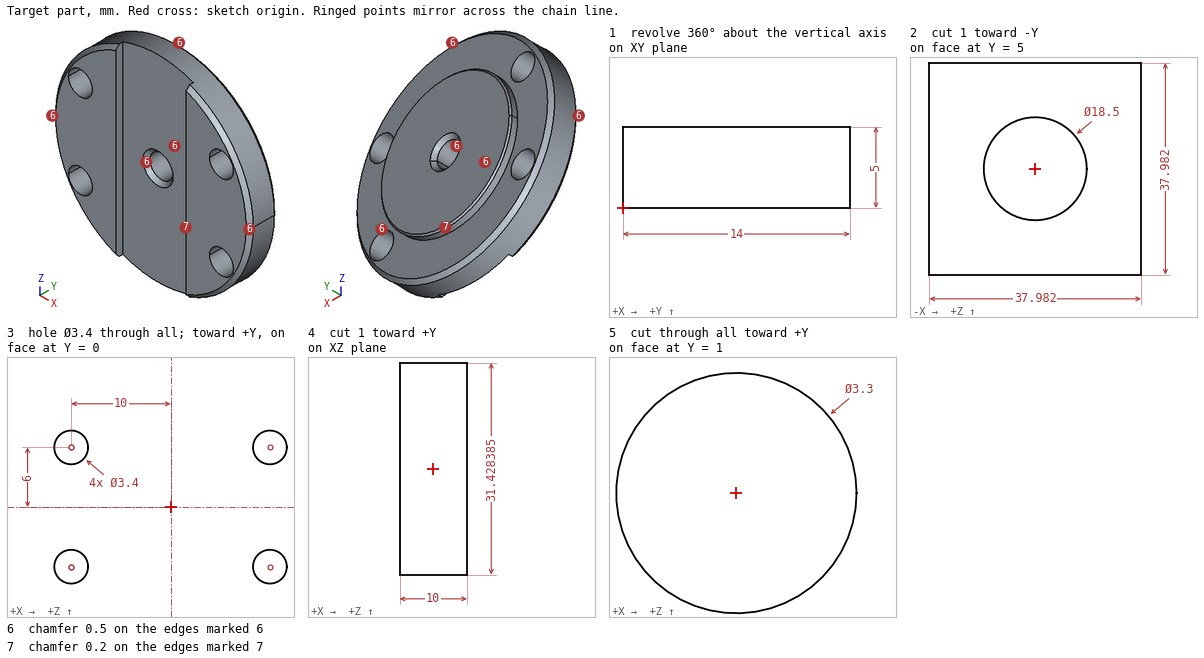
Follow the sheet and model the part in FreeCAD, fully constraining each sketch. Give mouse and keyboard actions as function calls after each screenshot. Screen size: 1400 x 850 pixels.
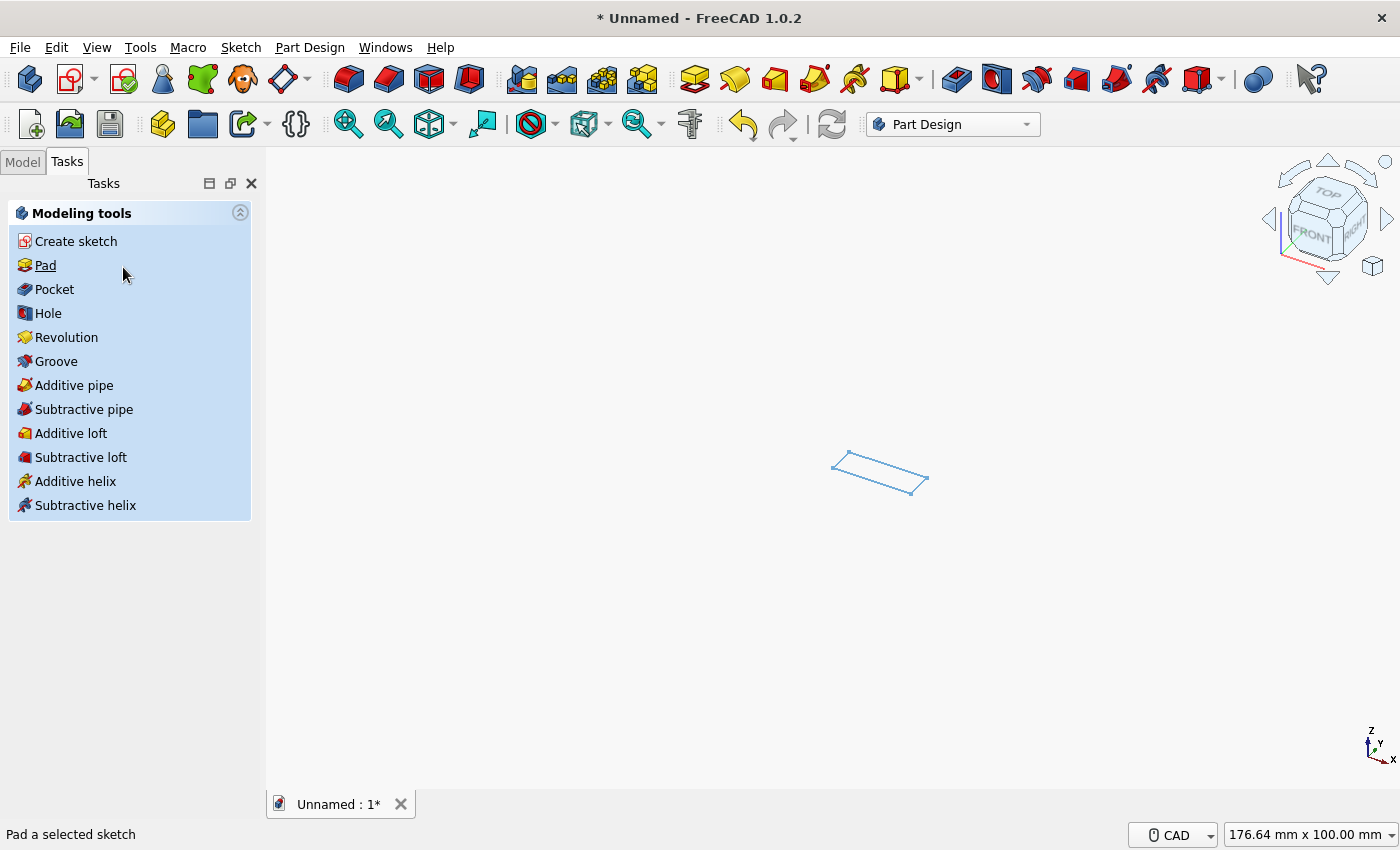
click(736, 80)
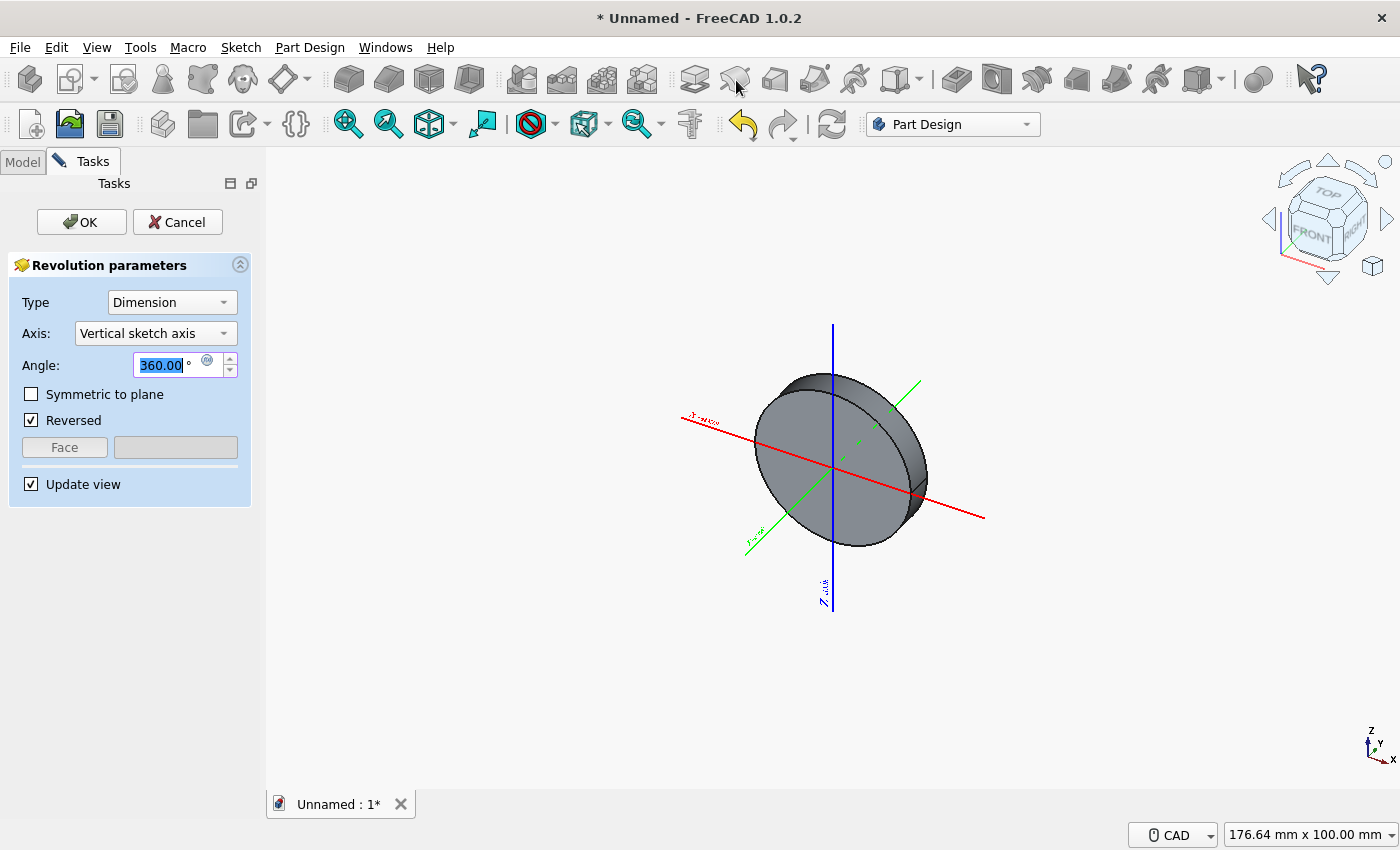
click(82, 222)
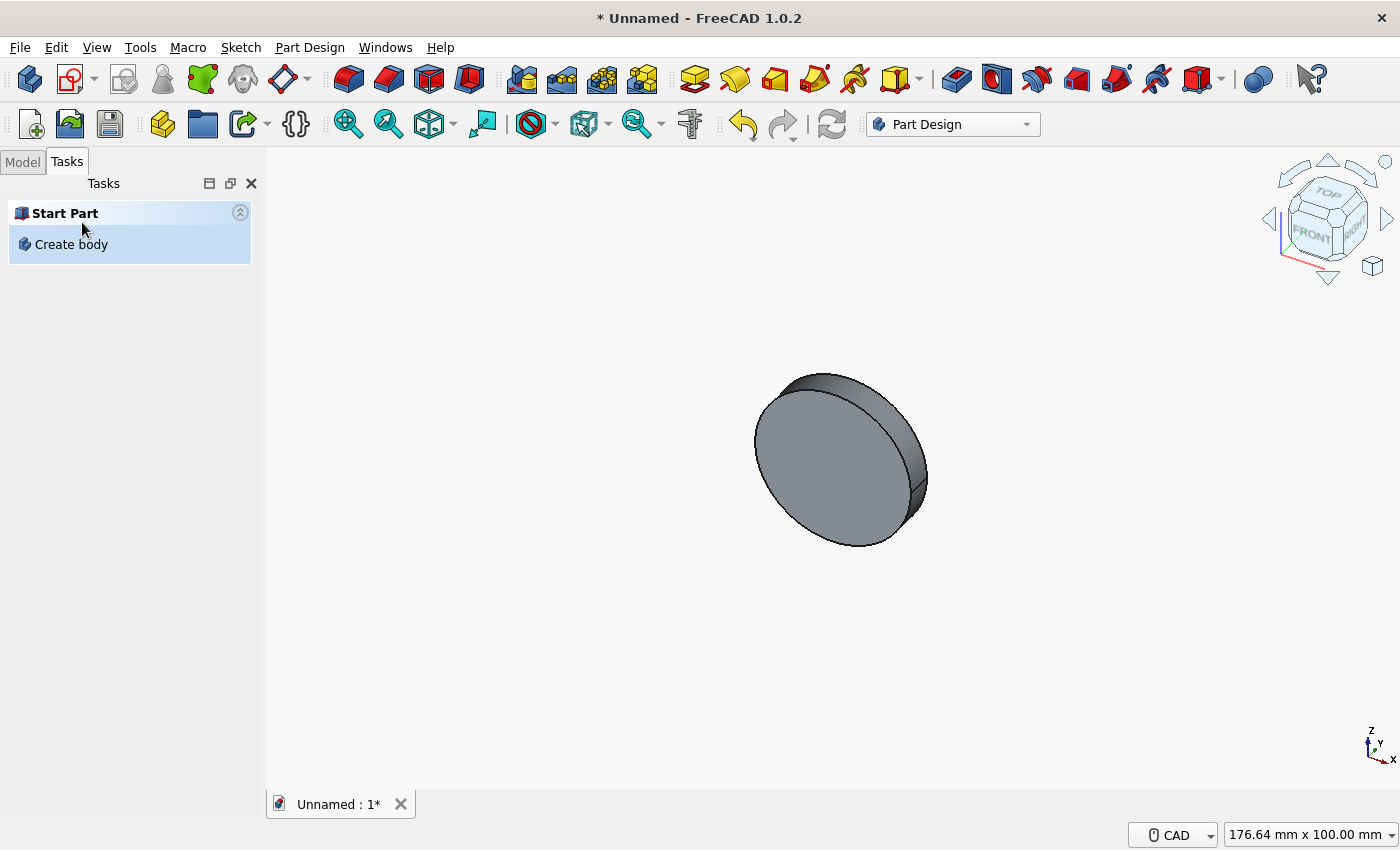
key(v)
key(f)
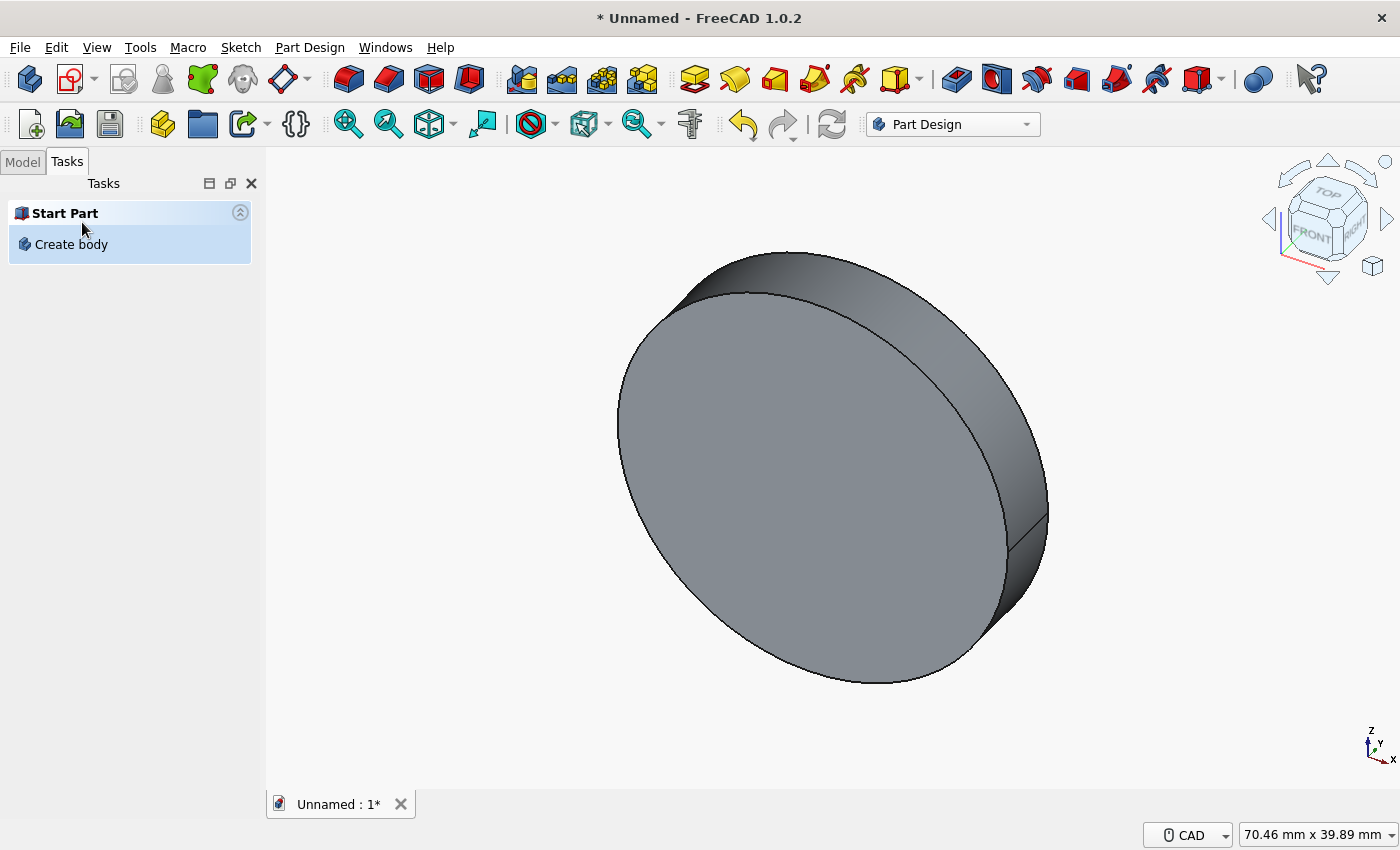
key(4)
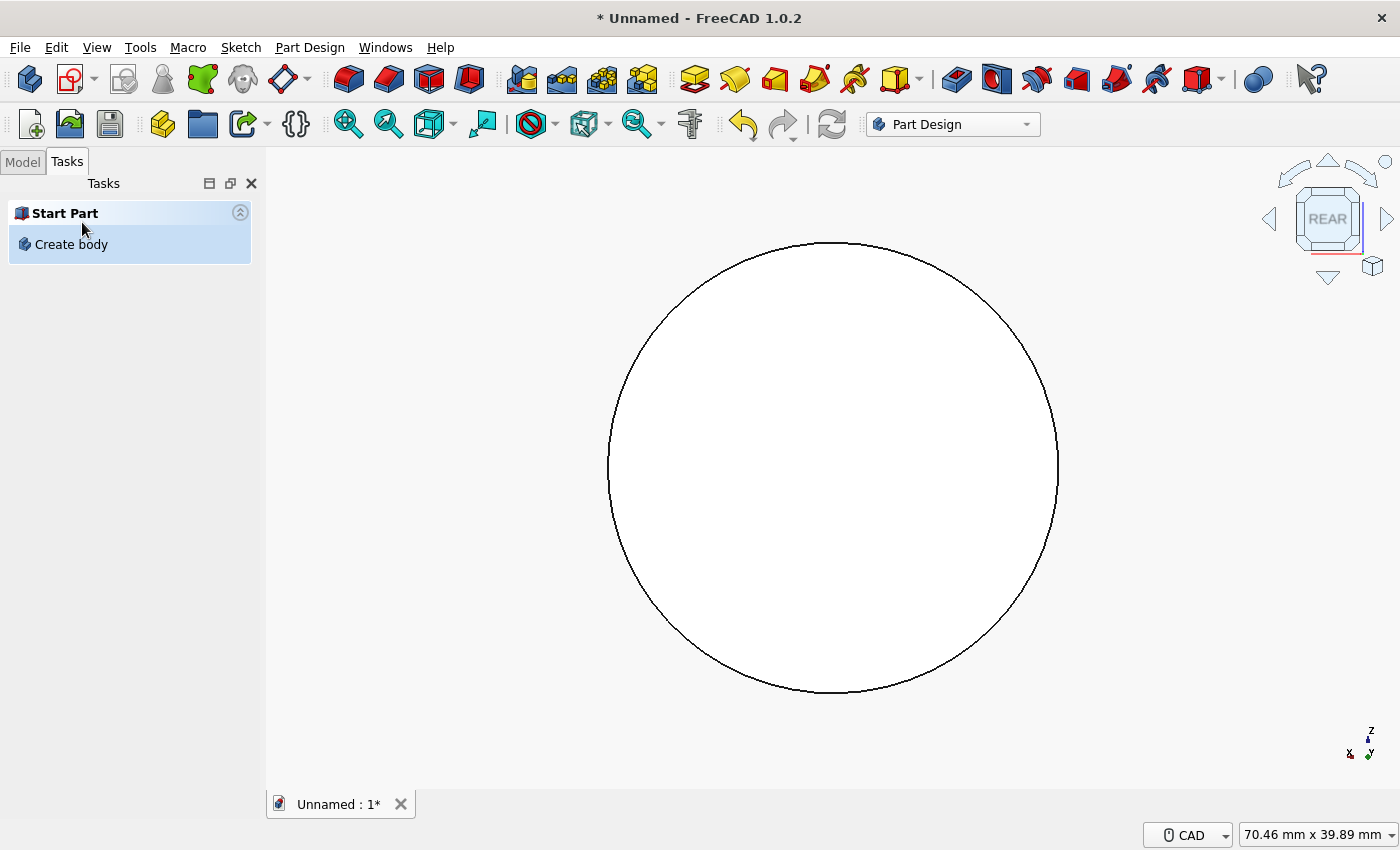
click(833, 467)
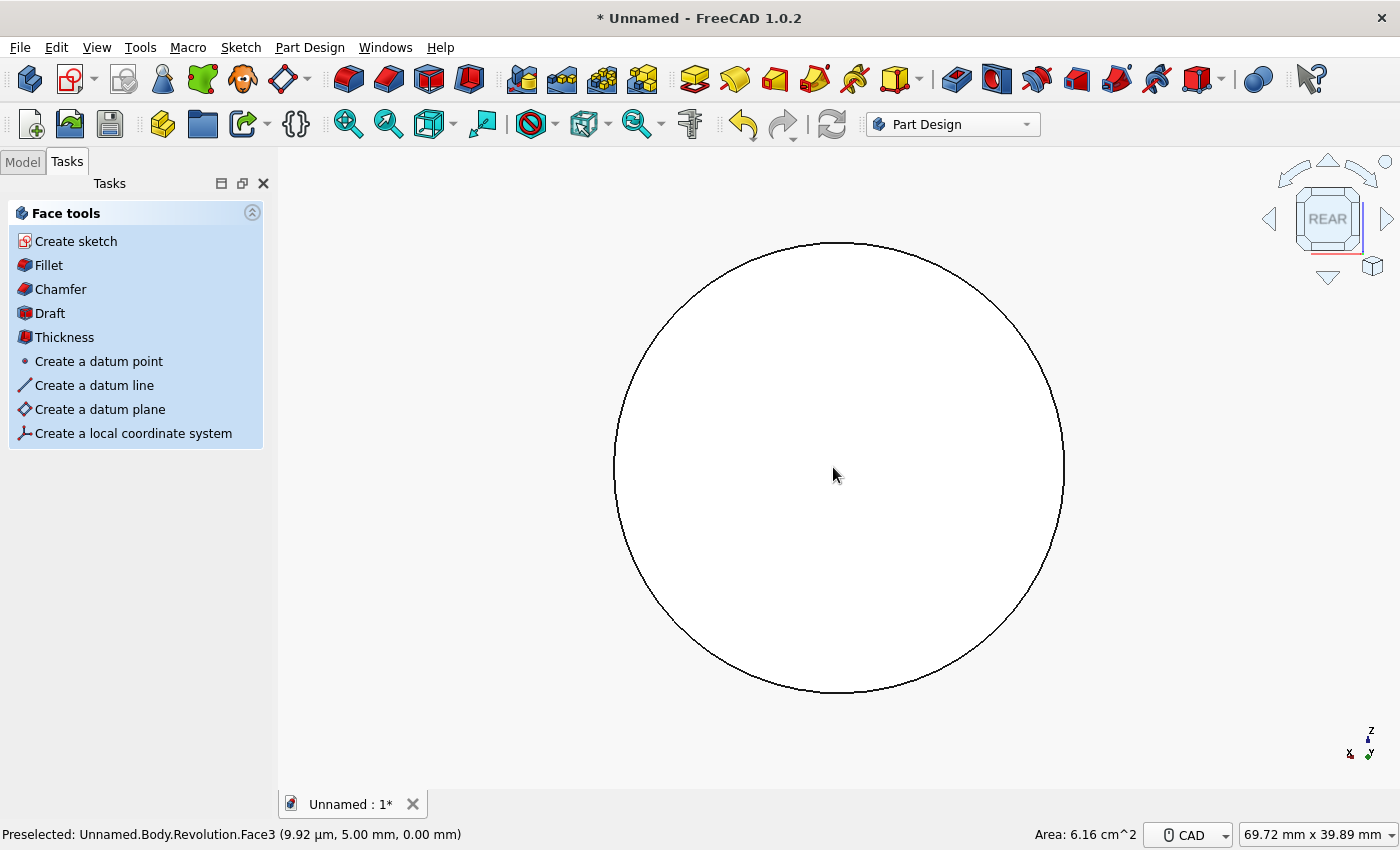
click(70, 80)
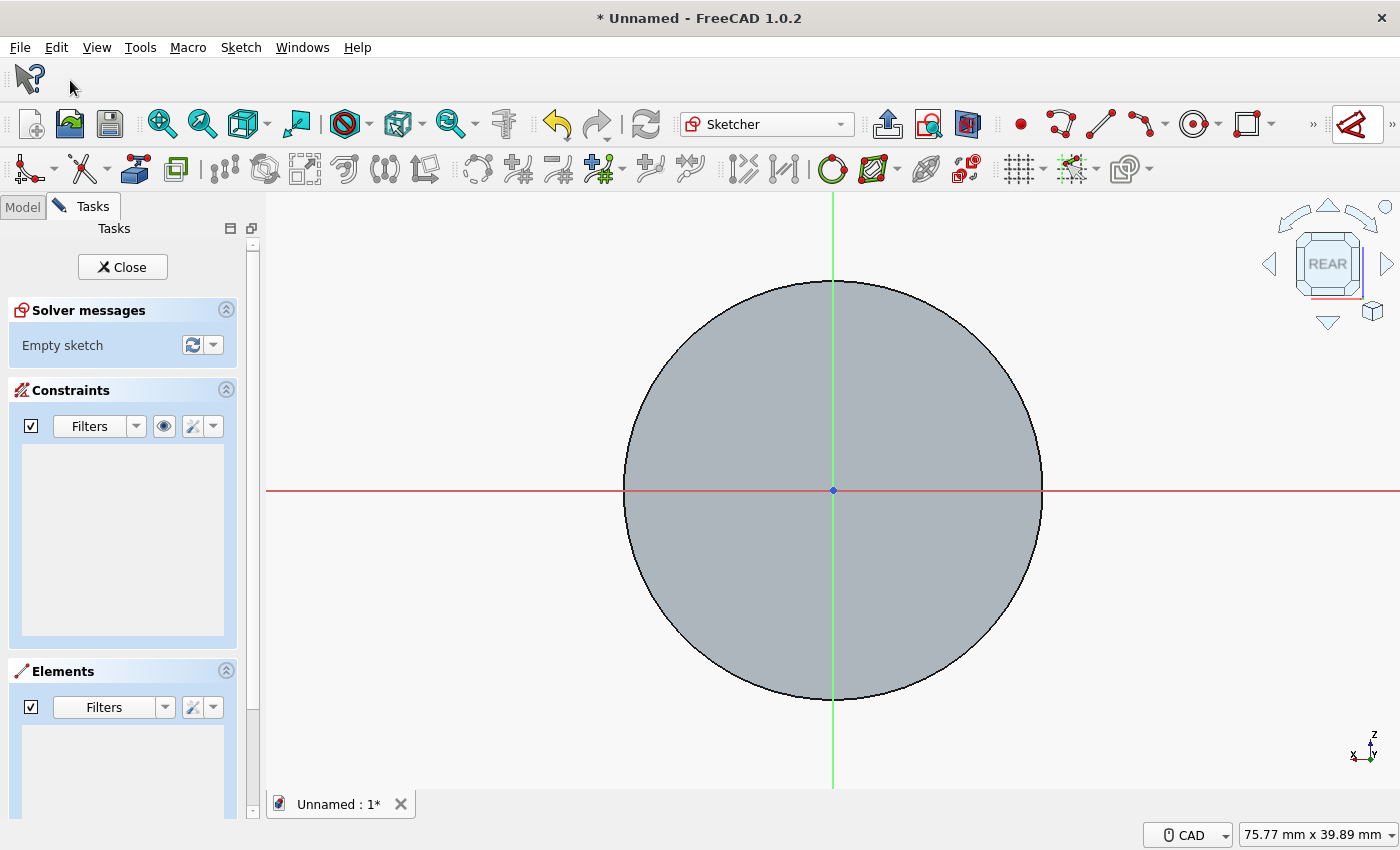
scroll(625, 491, down, 2)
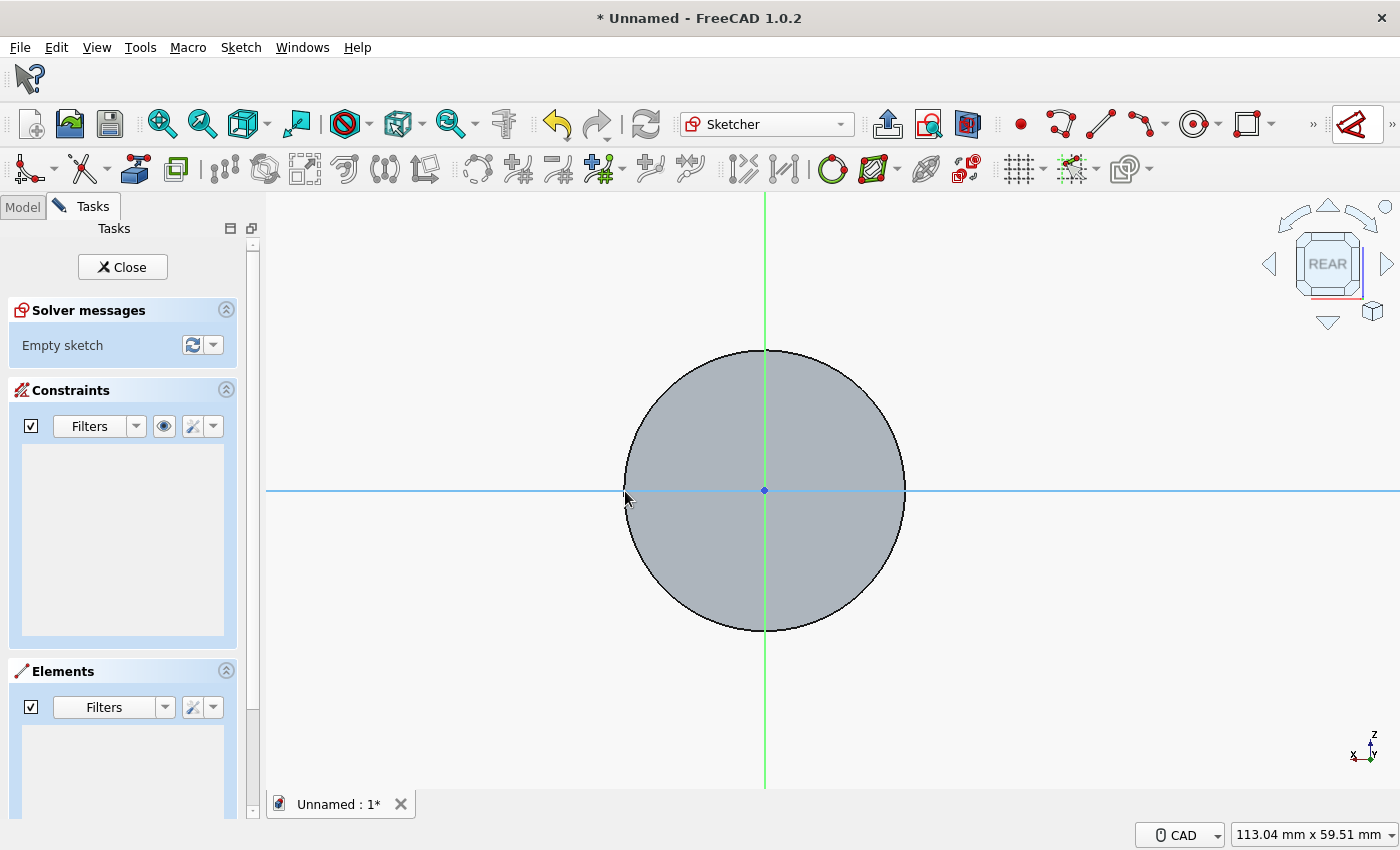
key(g)
key(v)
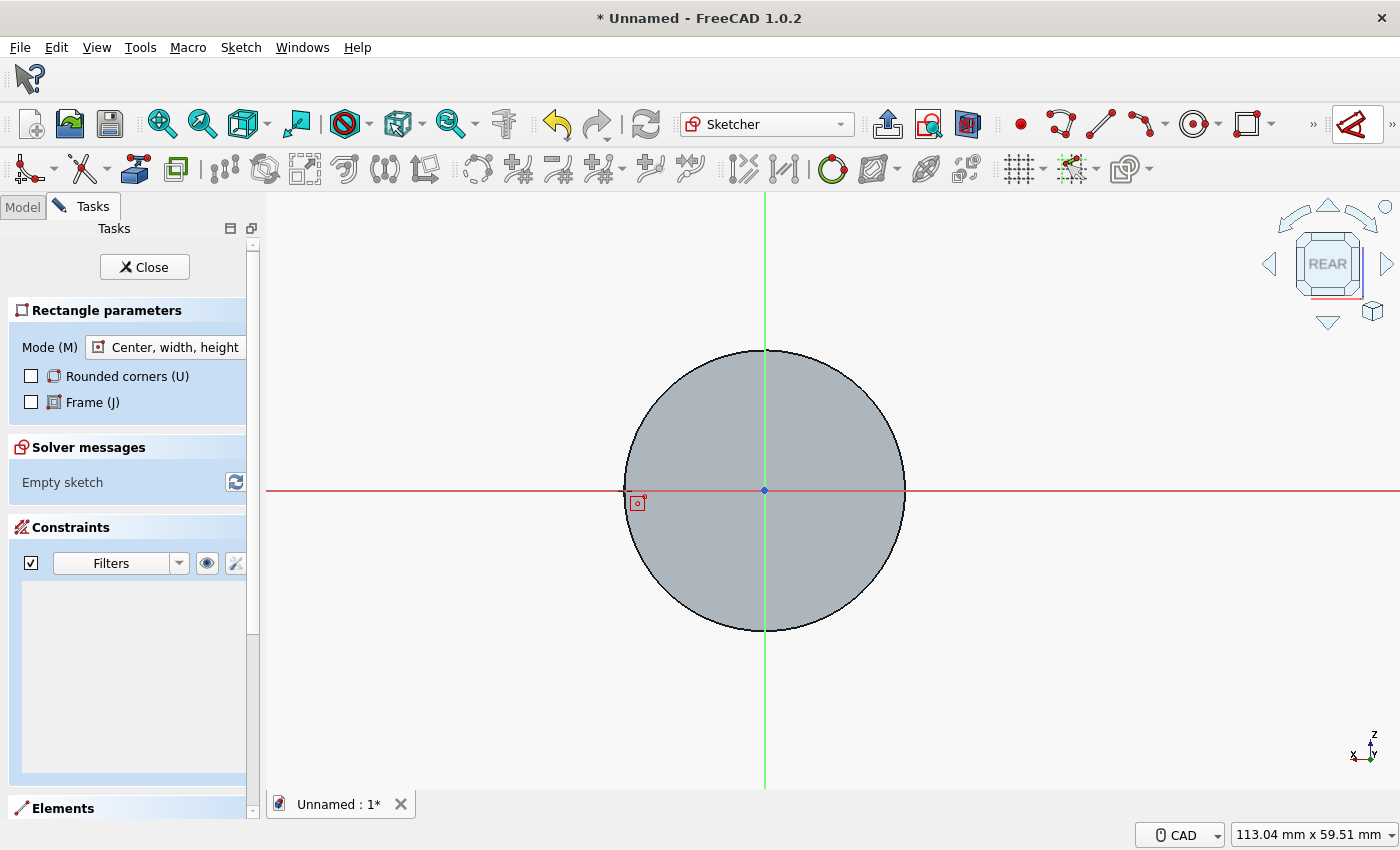
click(765, 491)
move(955, 300)